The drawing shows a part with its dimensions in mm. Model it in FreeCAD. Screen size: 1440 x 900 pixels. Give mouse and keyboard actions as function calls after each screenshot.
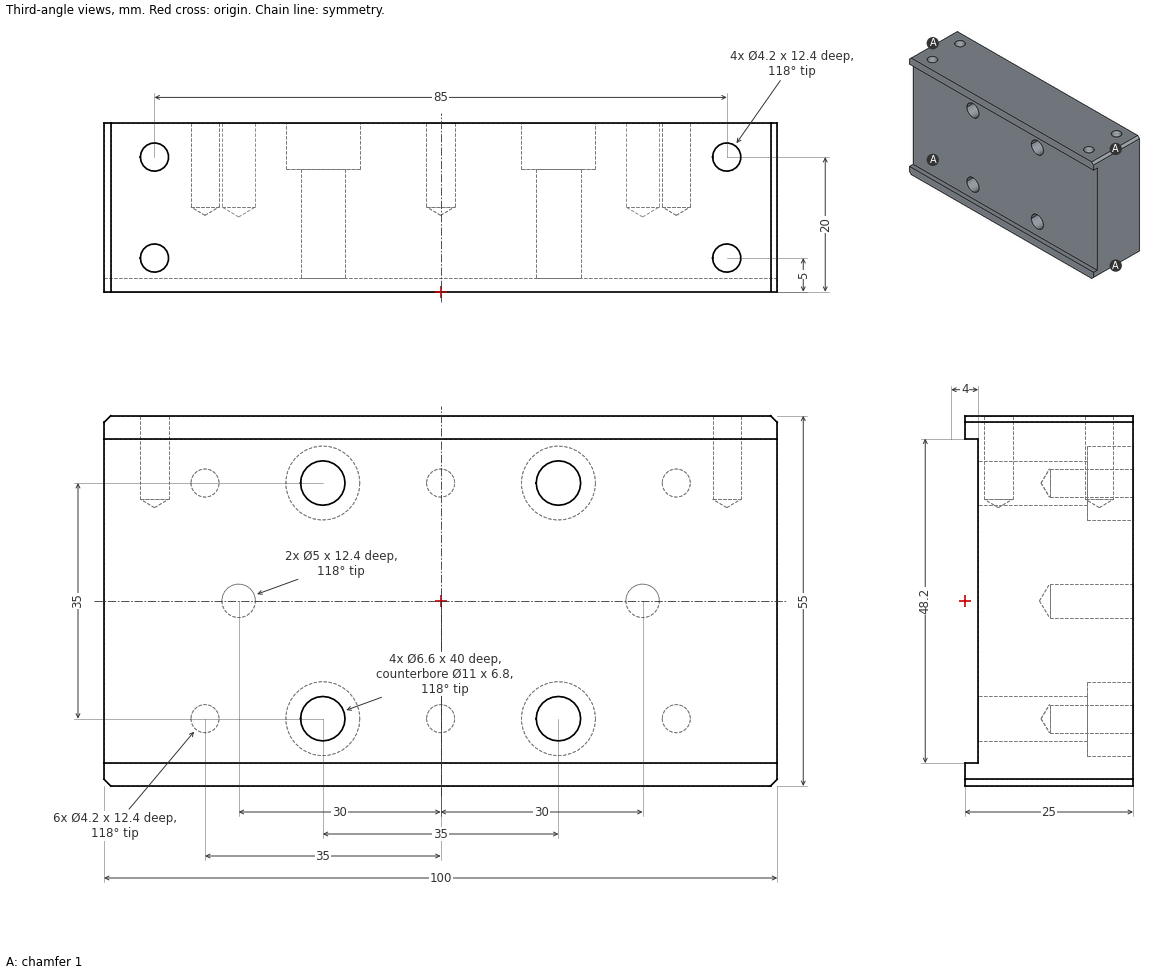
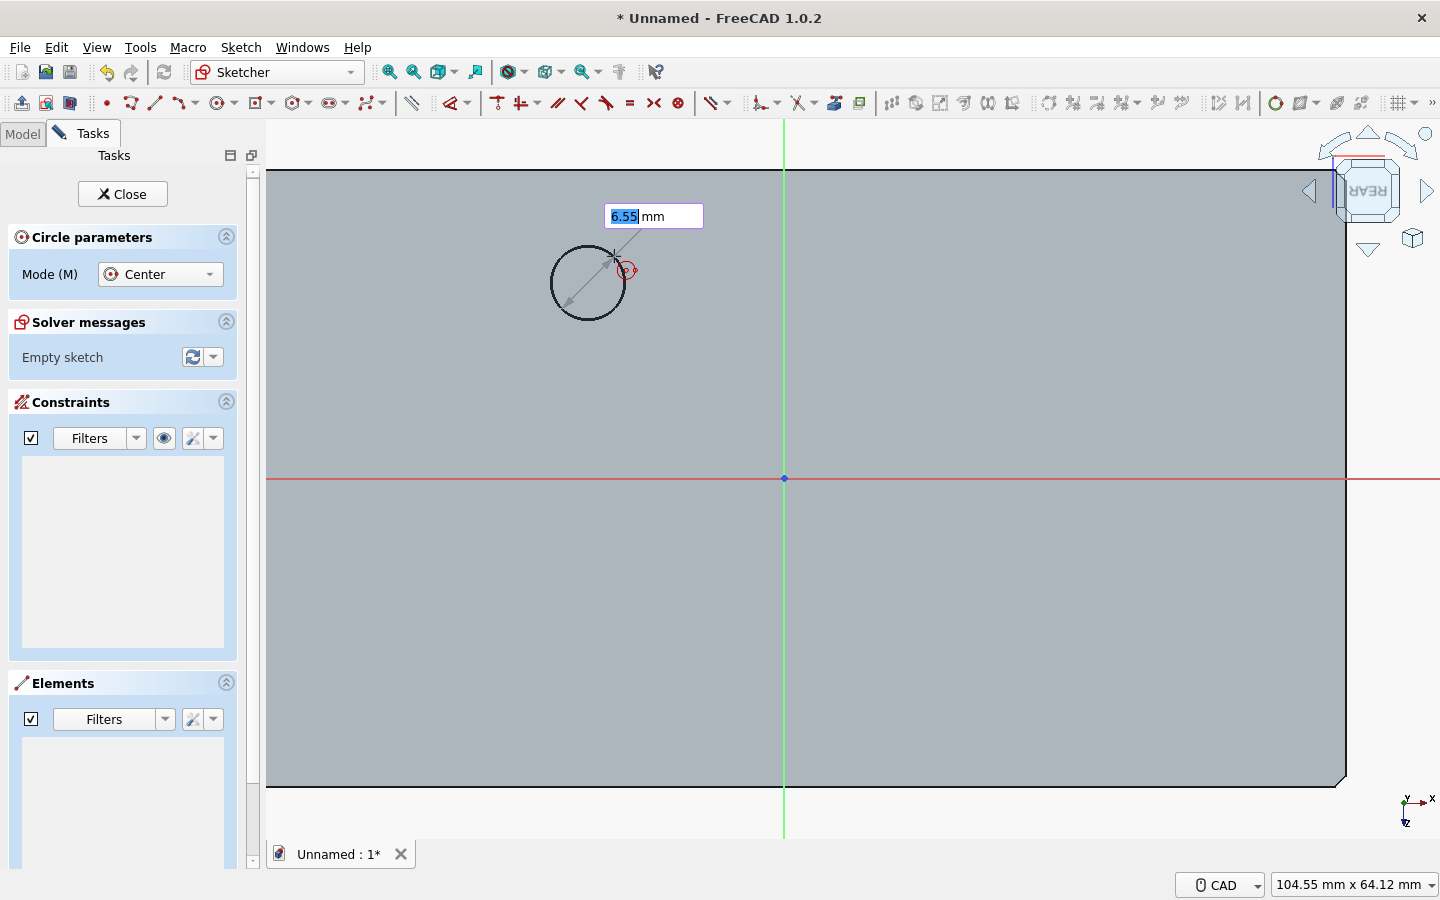
text(6.6)
key(Return)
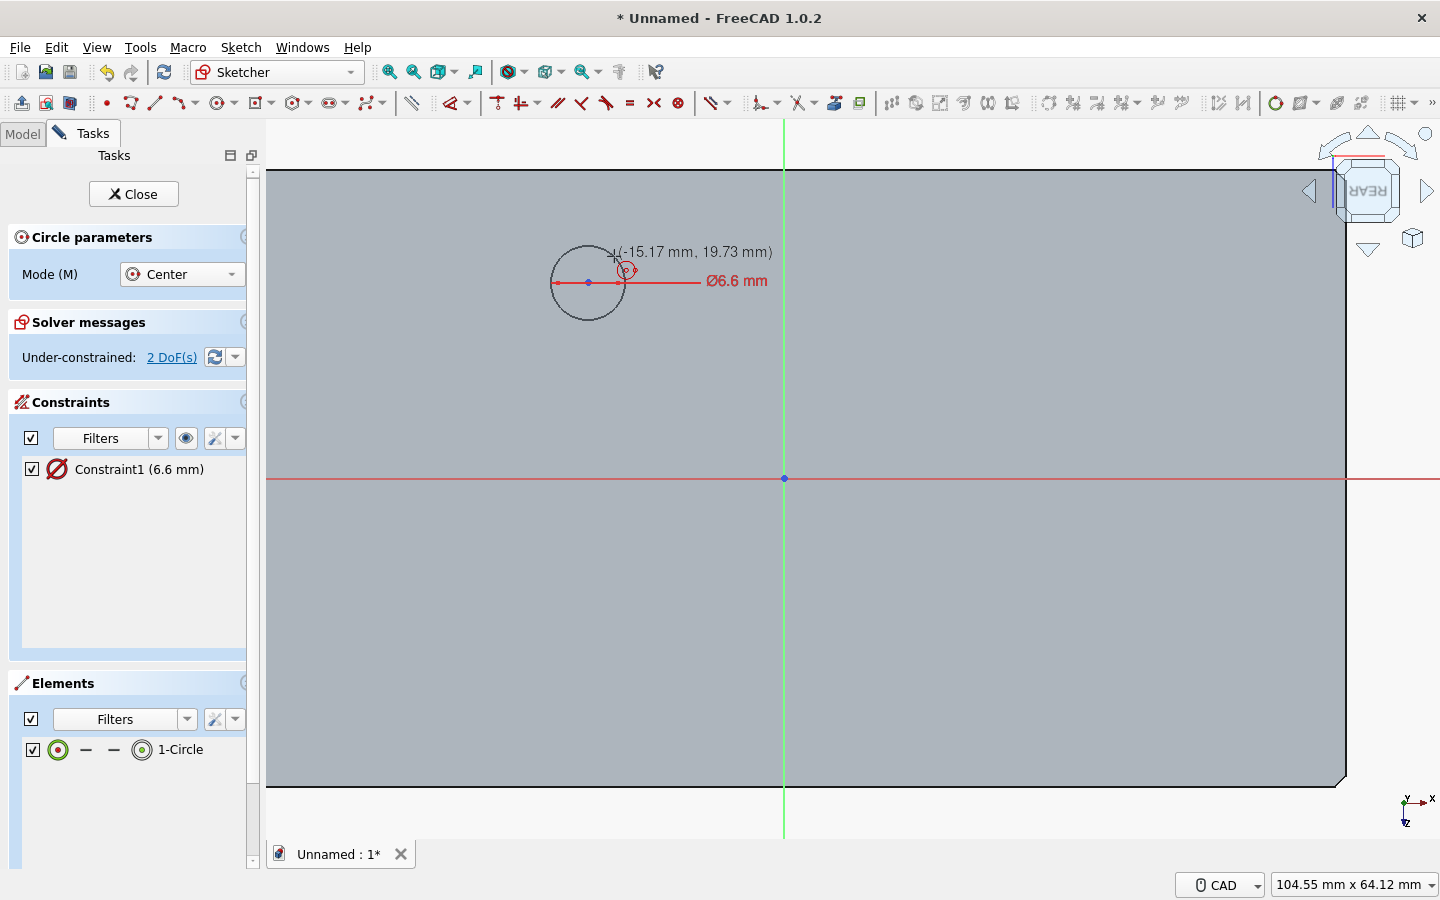
click(981, 282)
move(1007, 256)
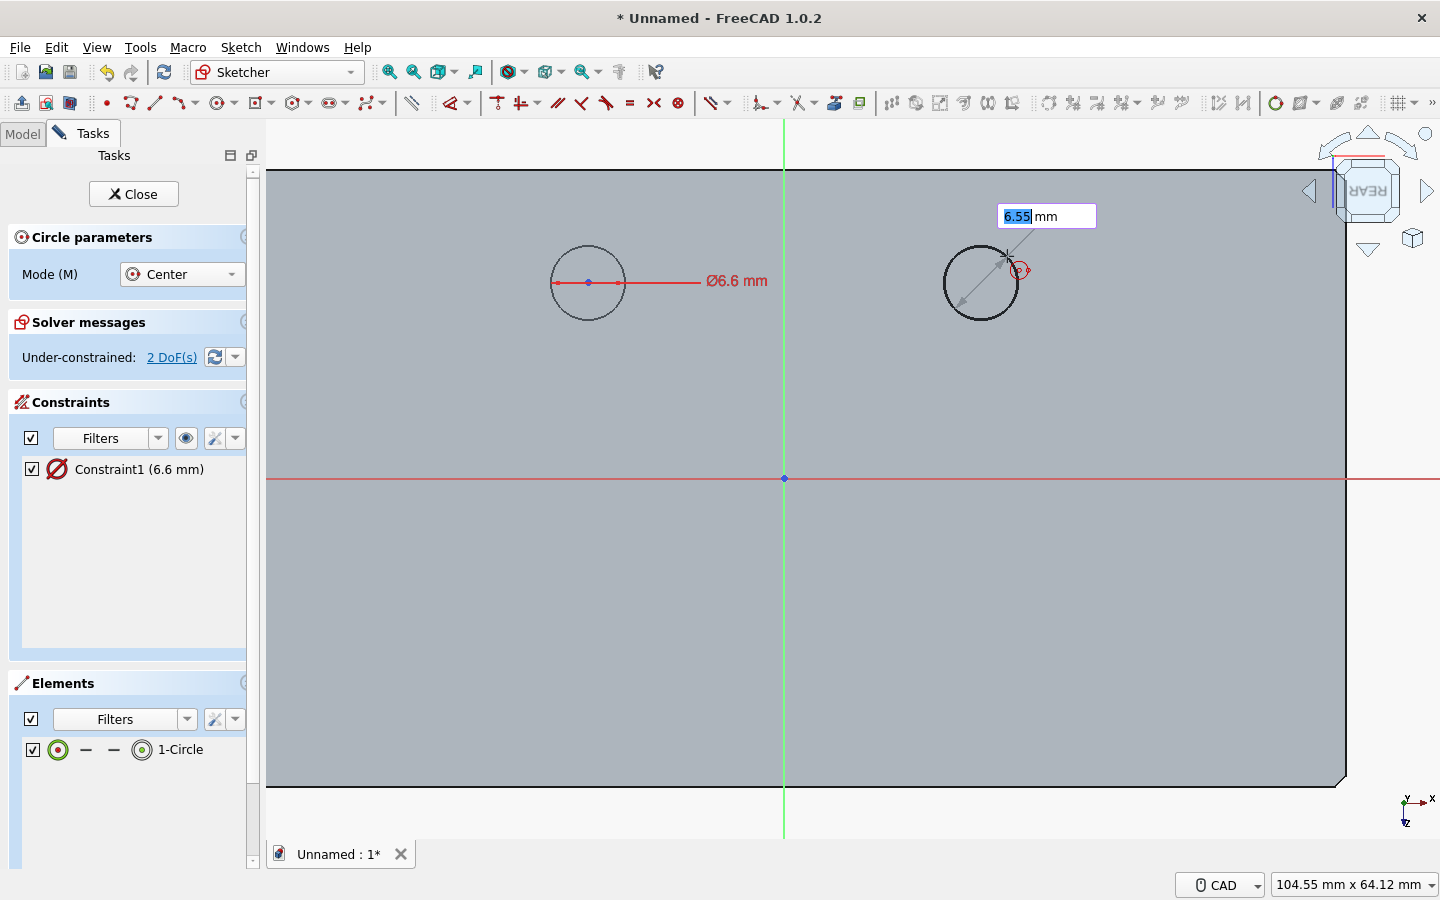
text(6.6)
key(Return)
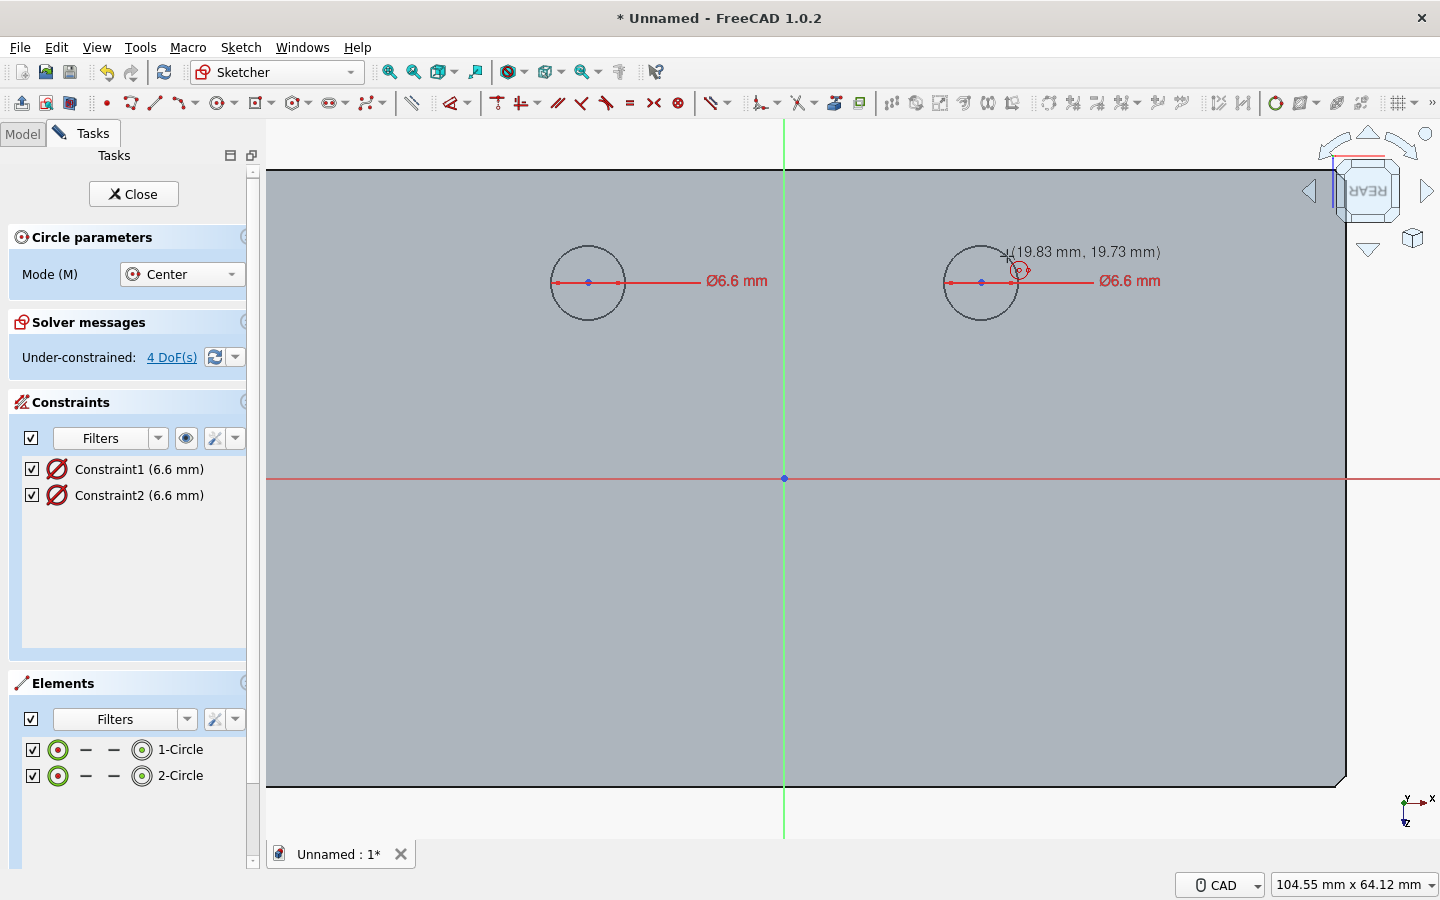
click(588, 675)
move(614, 649)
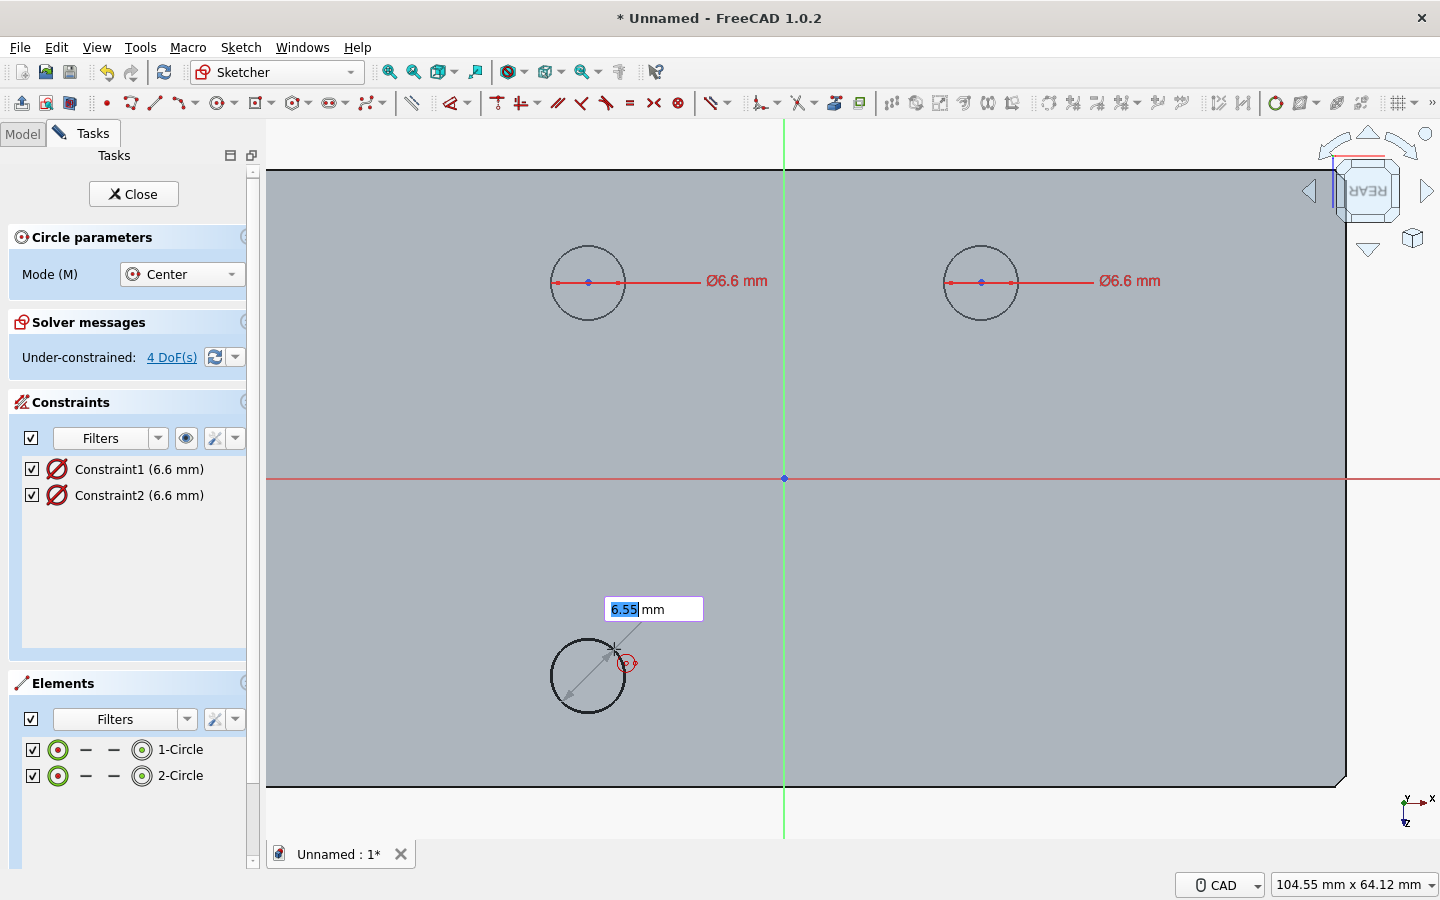
text(6.6)
key(Return)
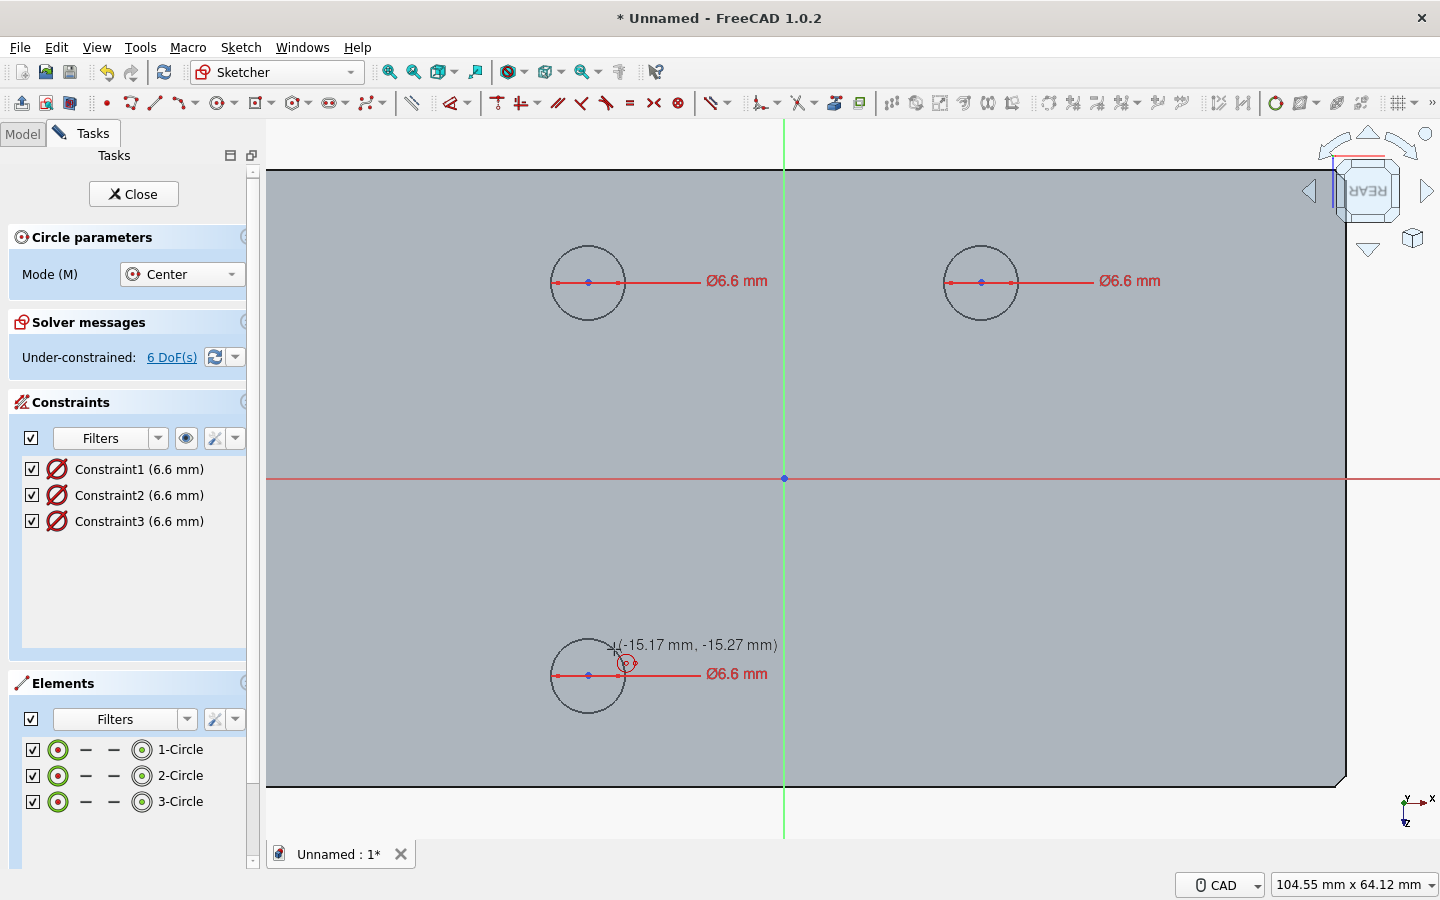
click(981, 675)
move(1007, 649)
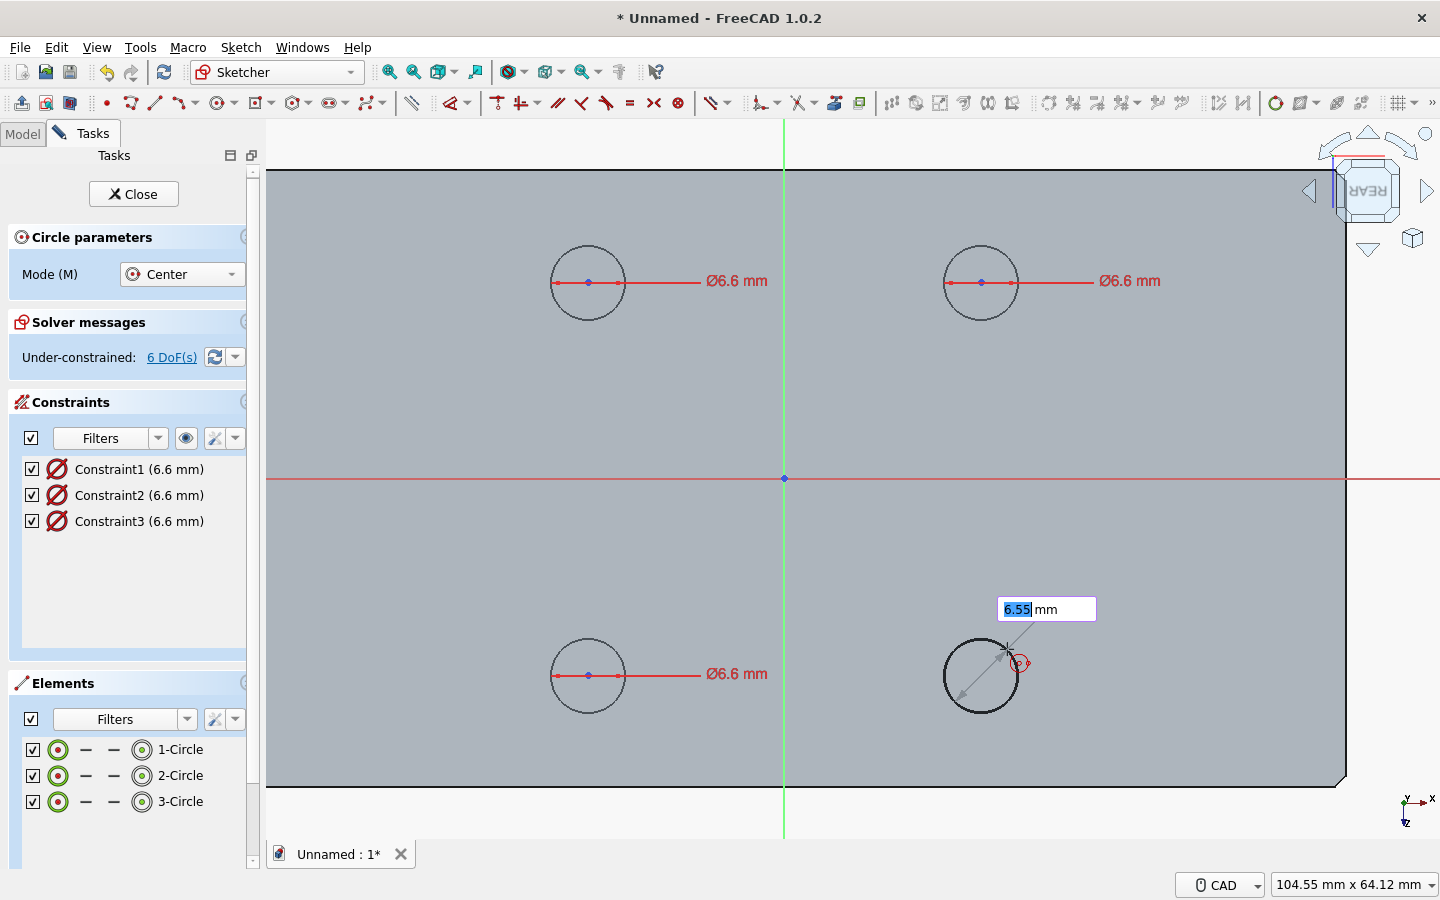
text(6.6)
key(Return)
key(Escape)